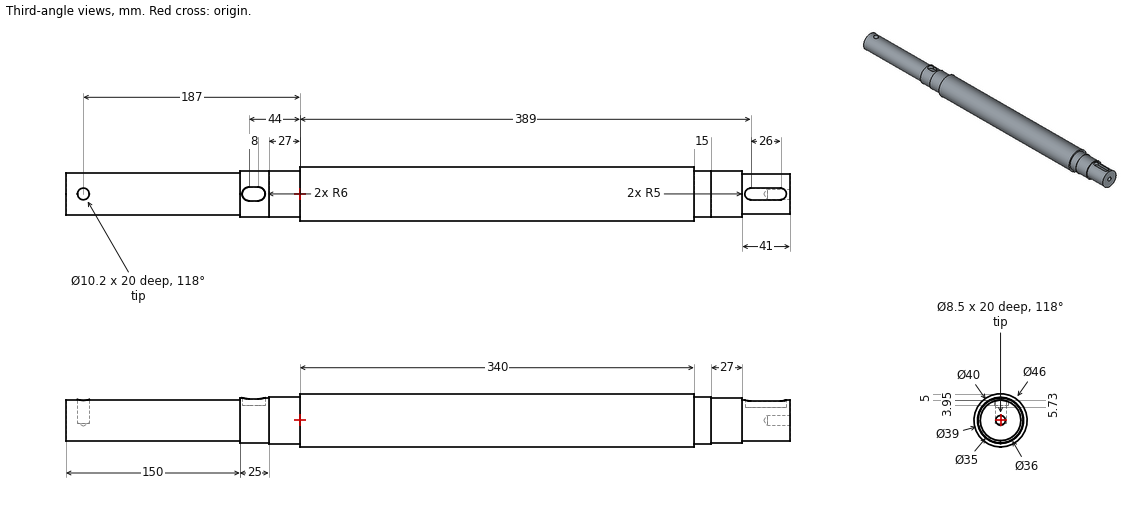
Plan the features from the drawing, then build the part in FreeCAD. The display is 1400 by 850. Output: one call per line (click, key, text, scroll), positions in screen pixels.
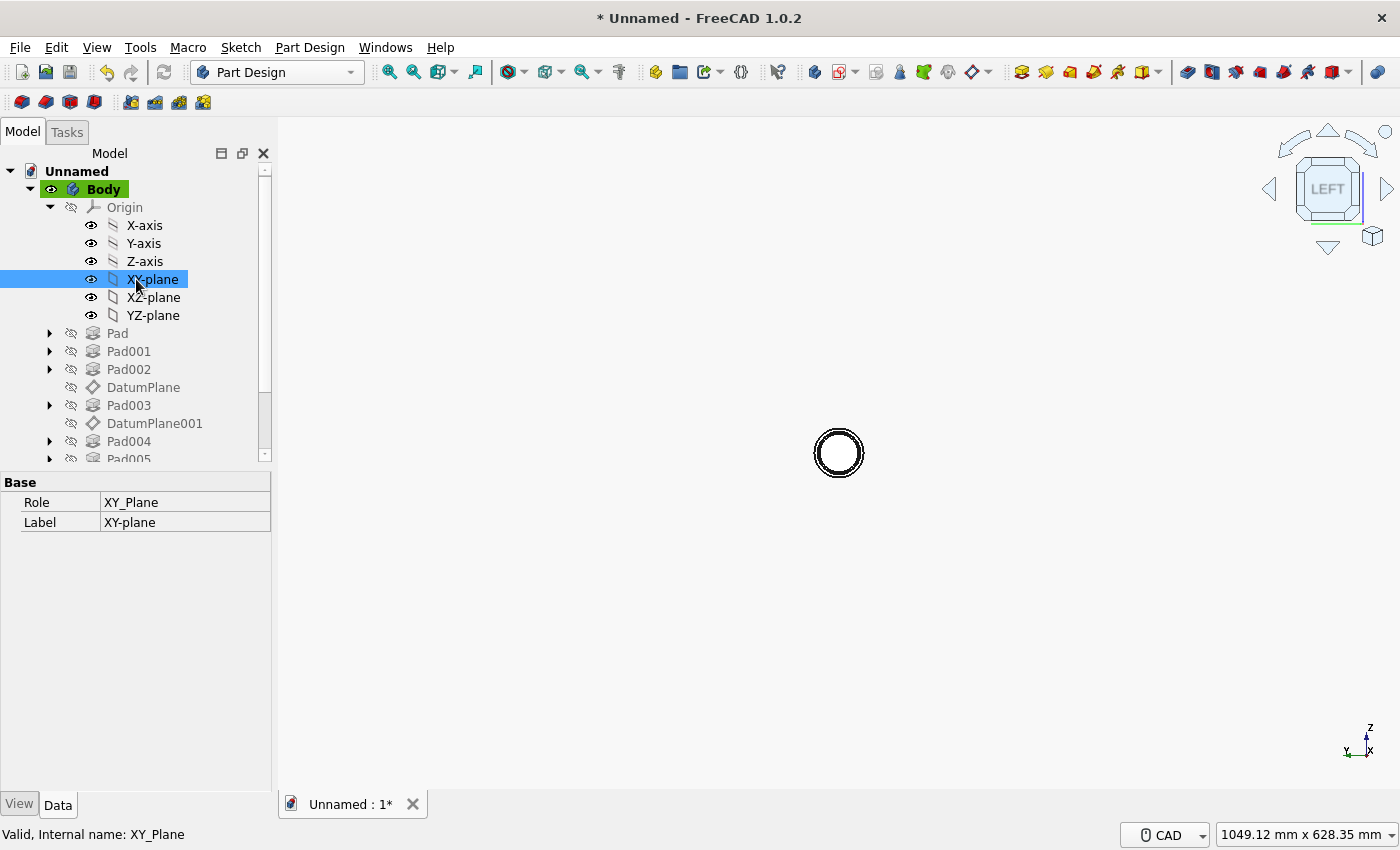
click(972, 72)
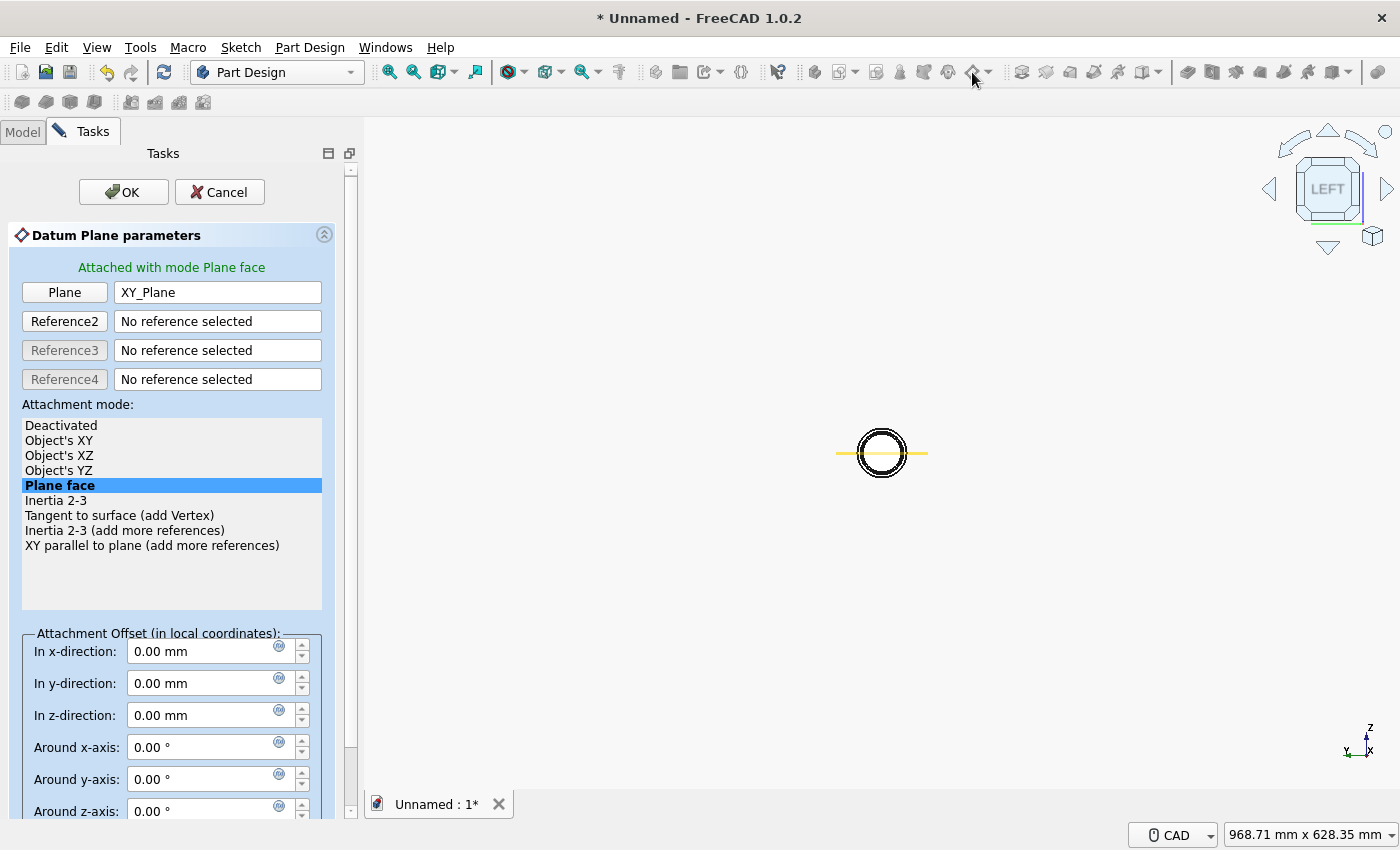
triple_click(210, 715)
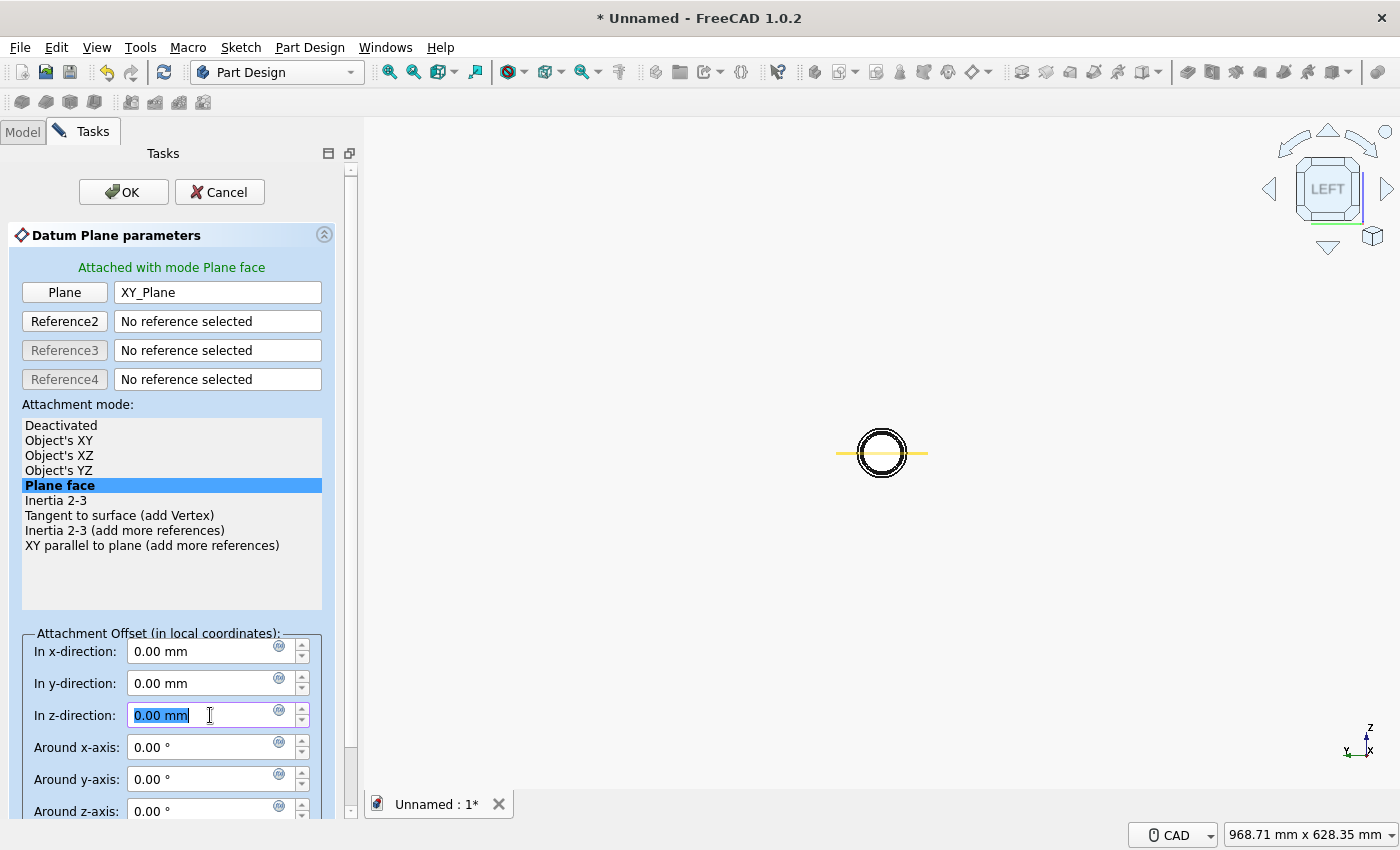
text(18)
key(Tab)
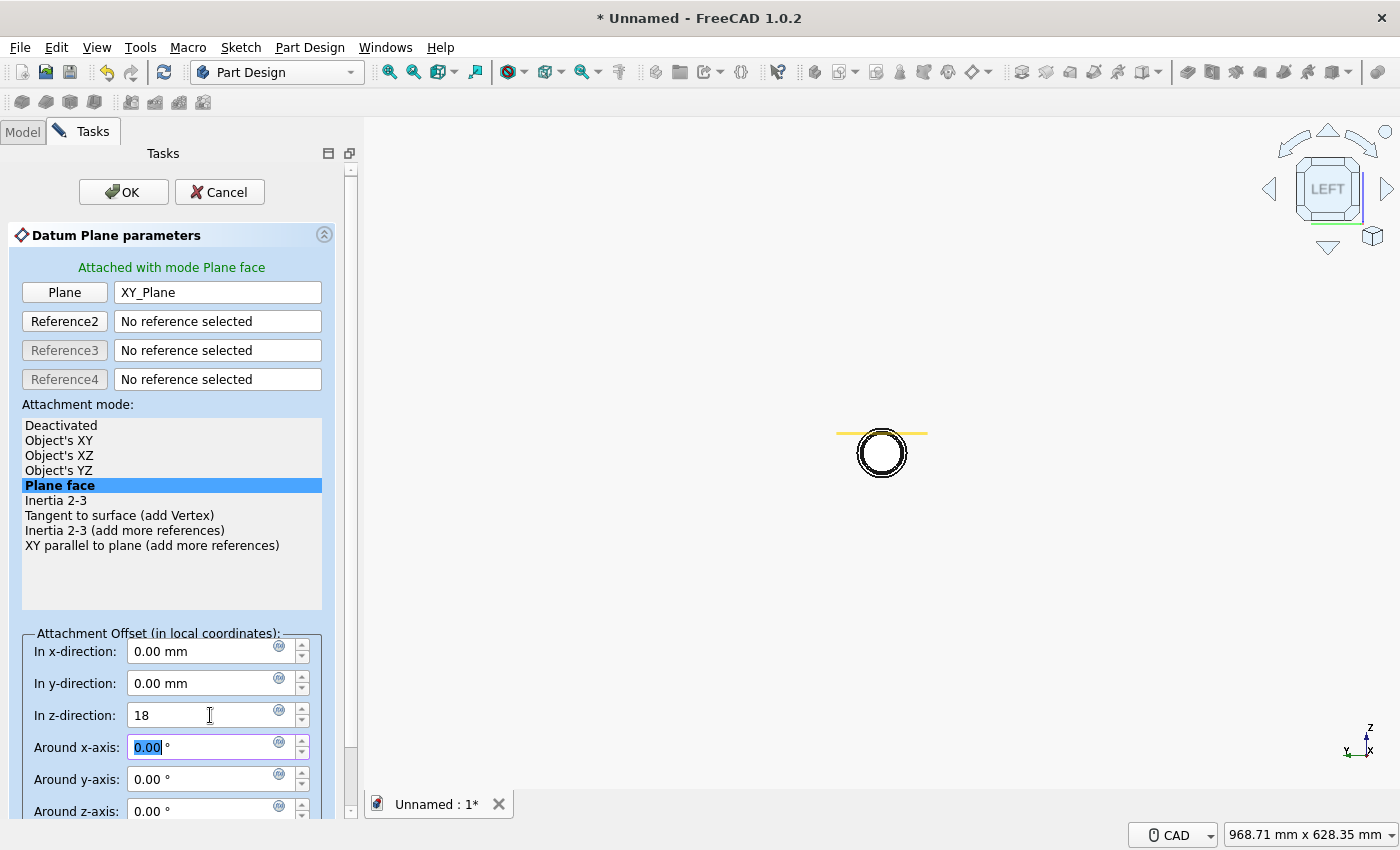
click(124, 192)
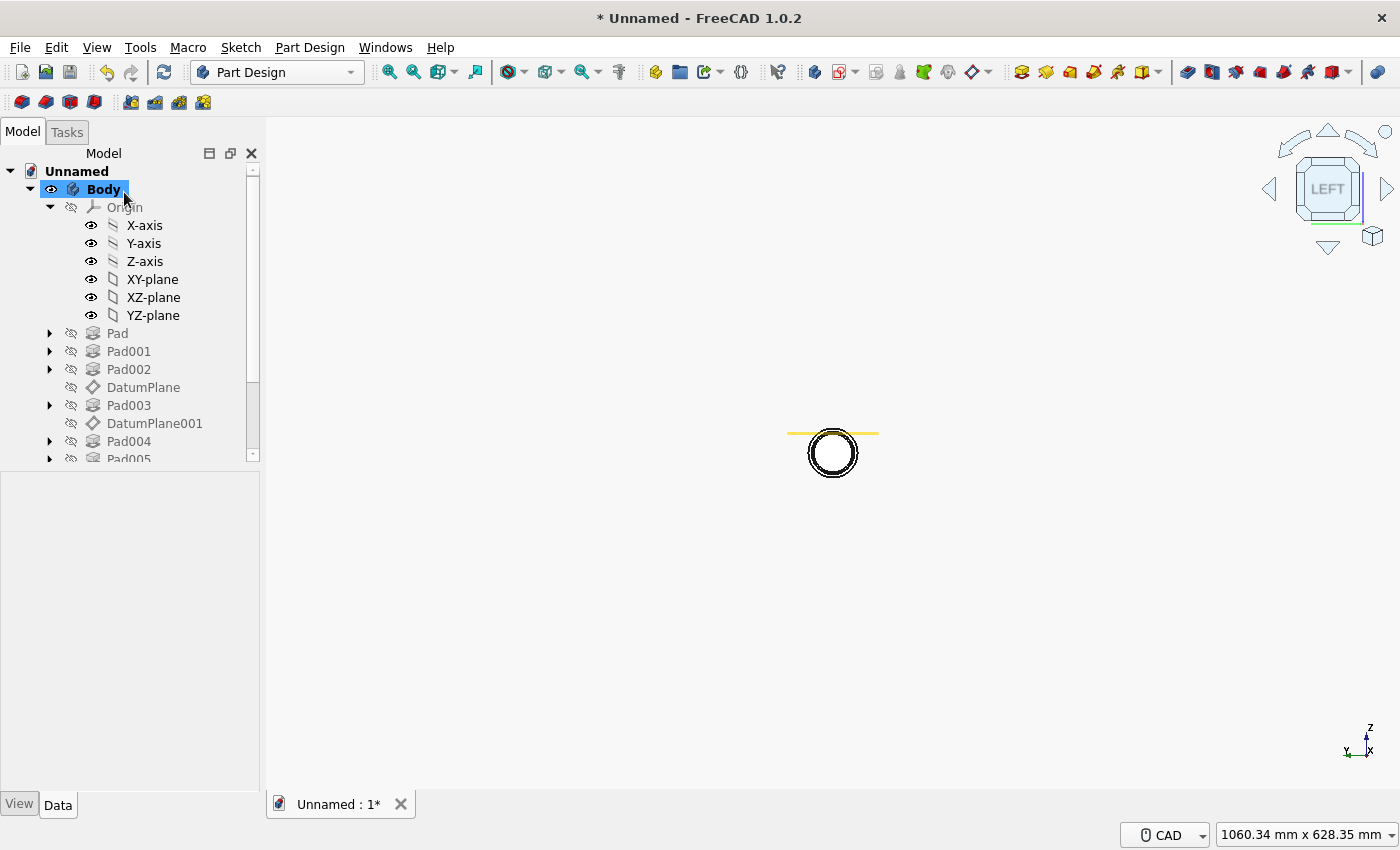
scroll(100, 311, down, 3)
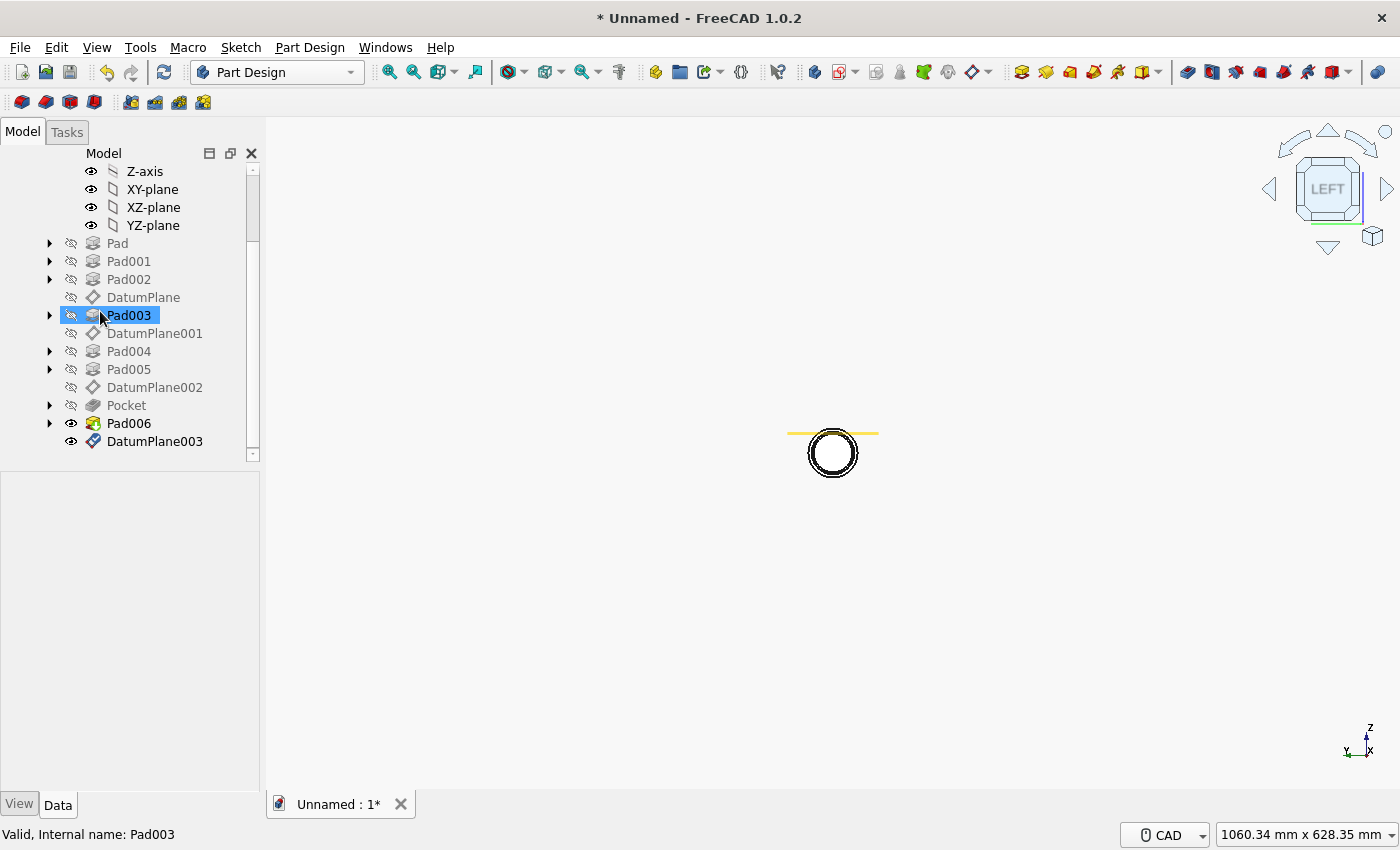
click(116, 441)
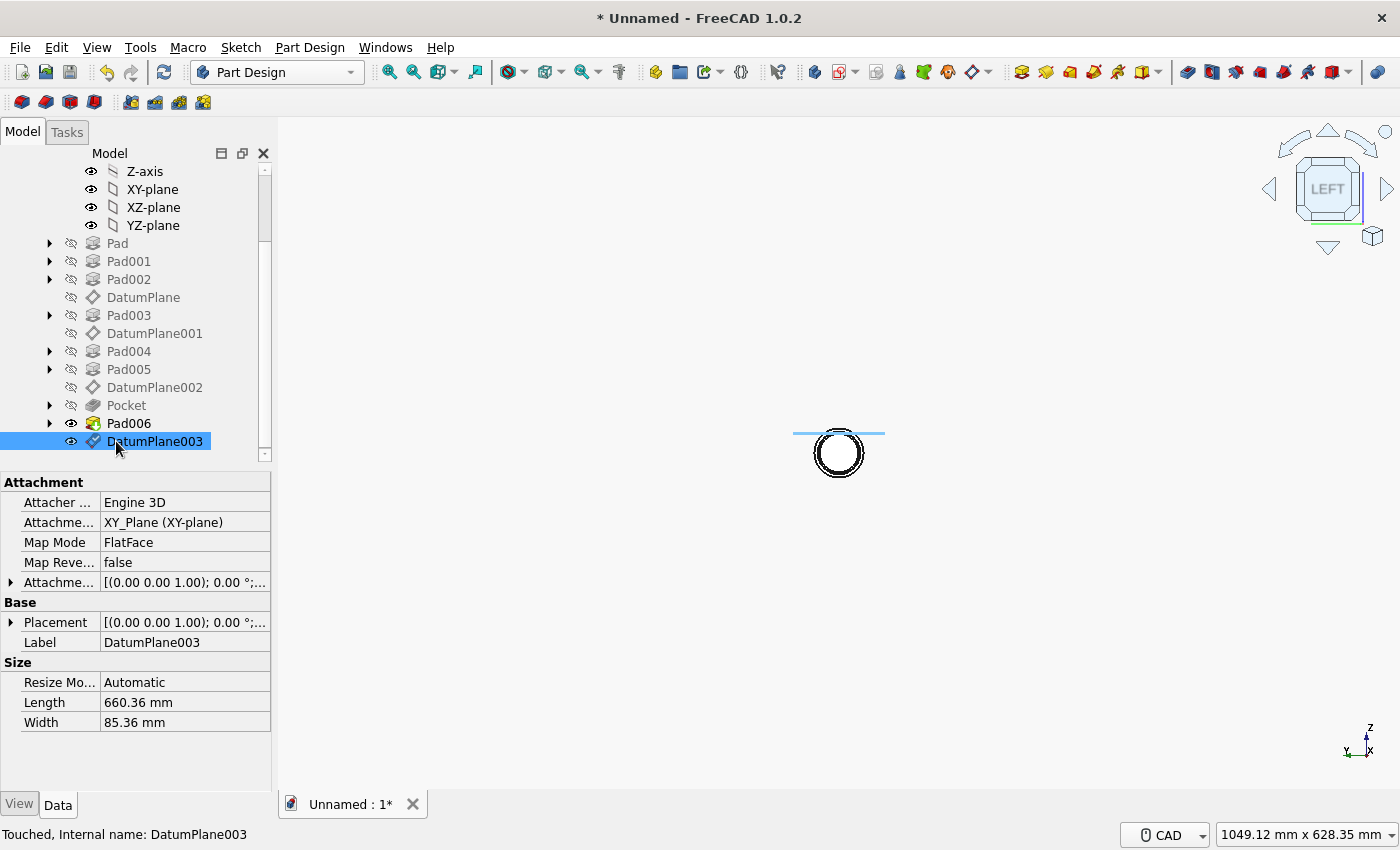
click(840, 72)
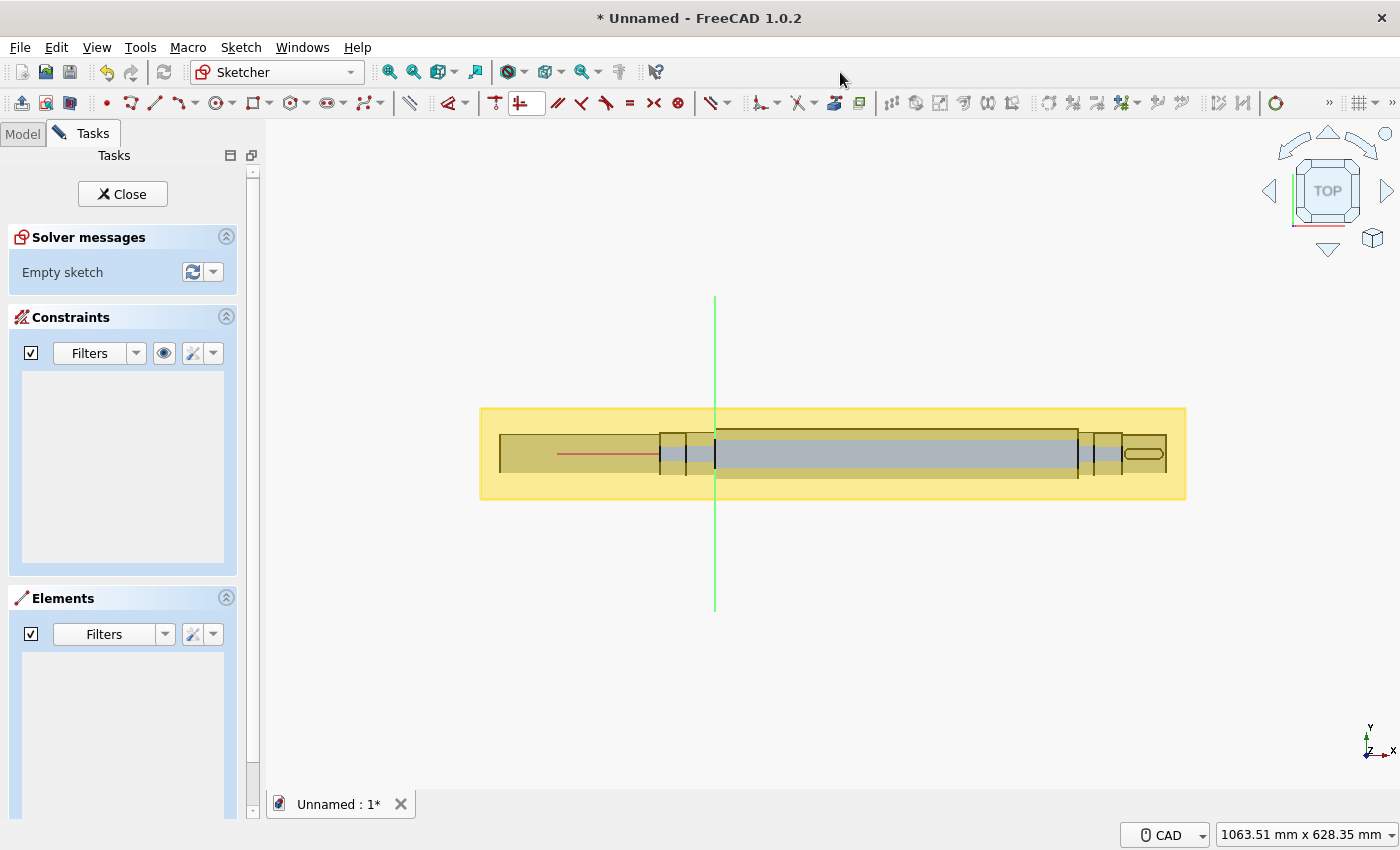
key(q)
key(s)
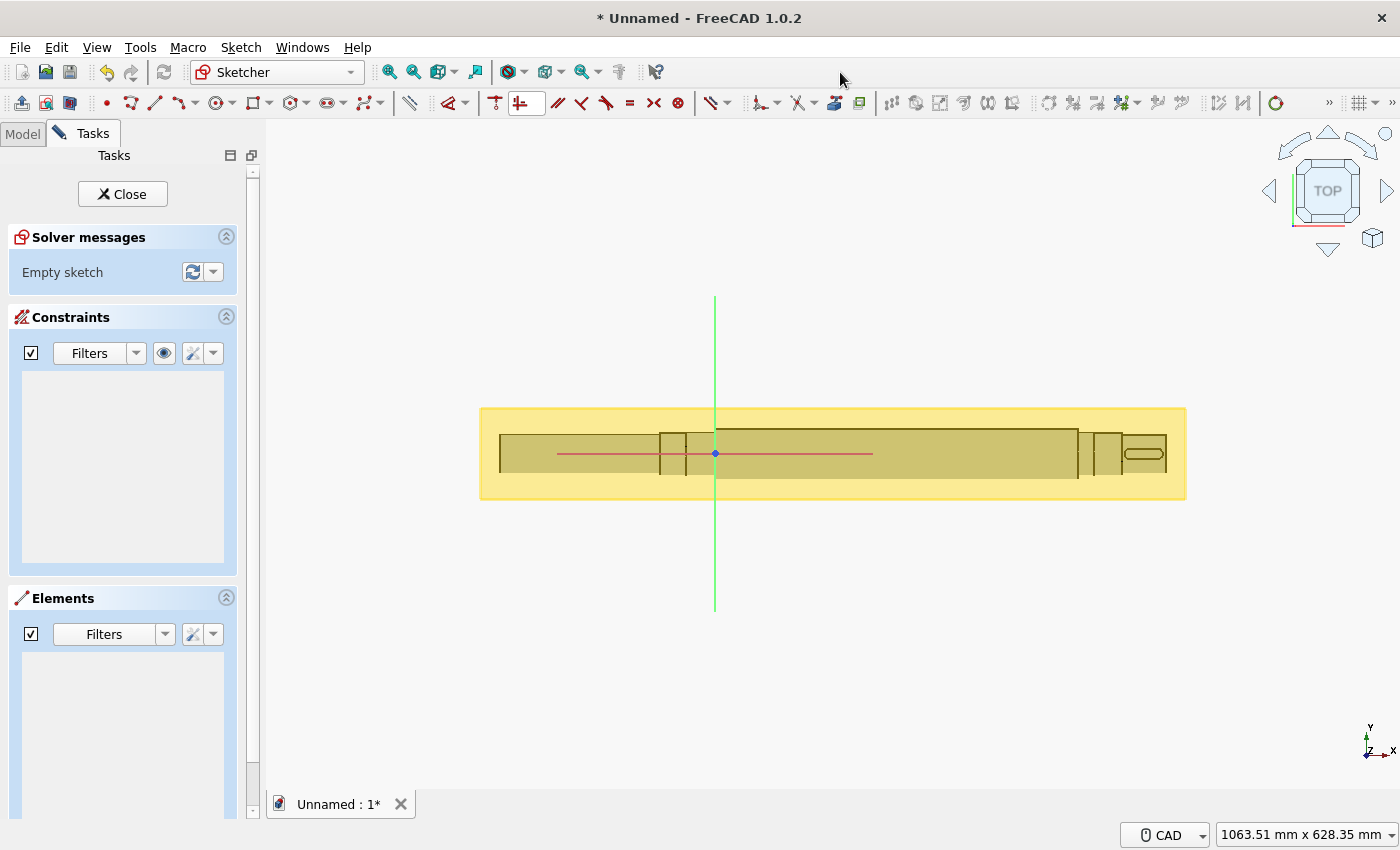
scroll(503, 454, up, 15)